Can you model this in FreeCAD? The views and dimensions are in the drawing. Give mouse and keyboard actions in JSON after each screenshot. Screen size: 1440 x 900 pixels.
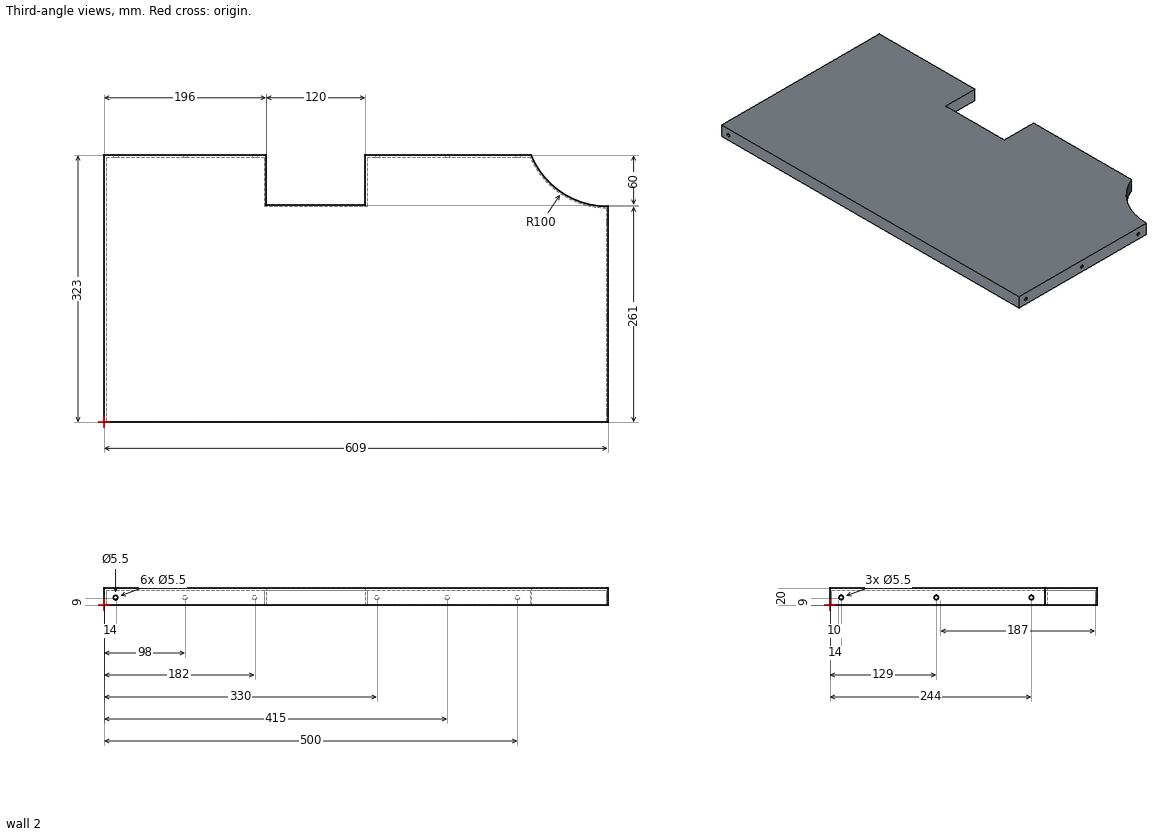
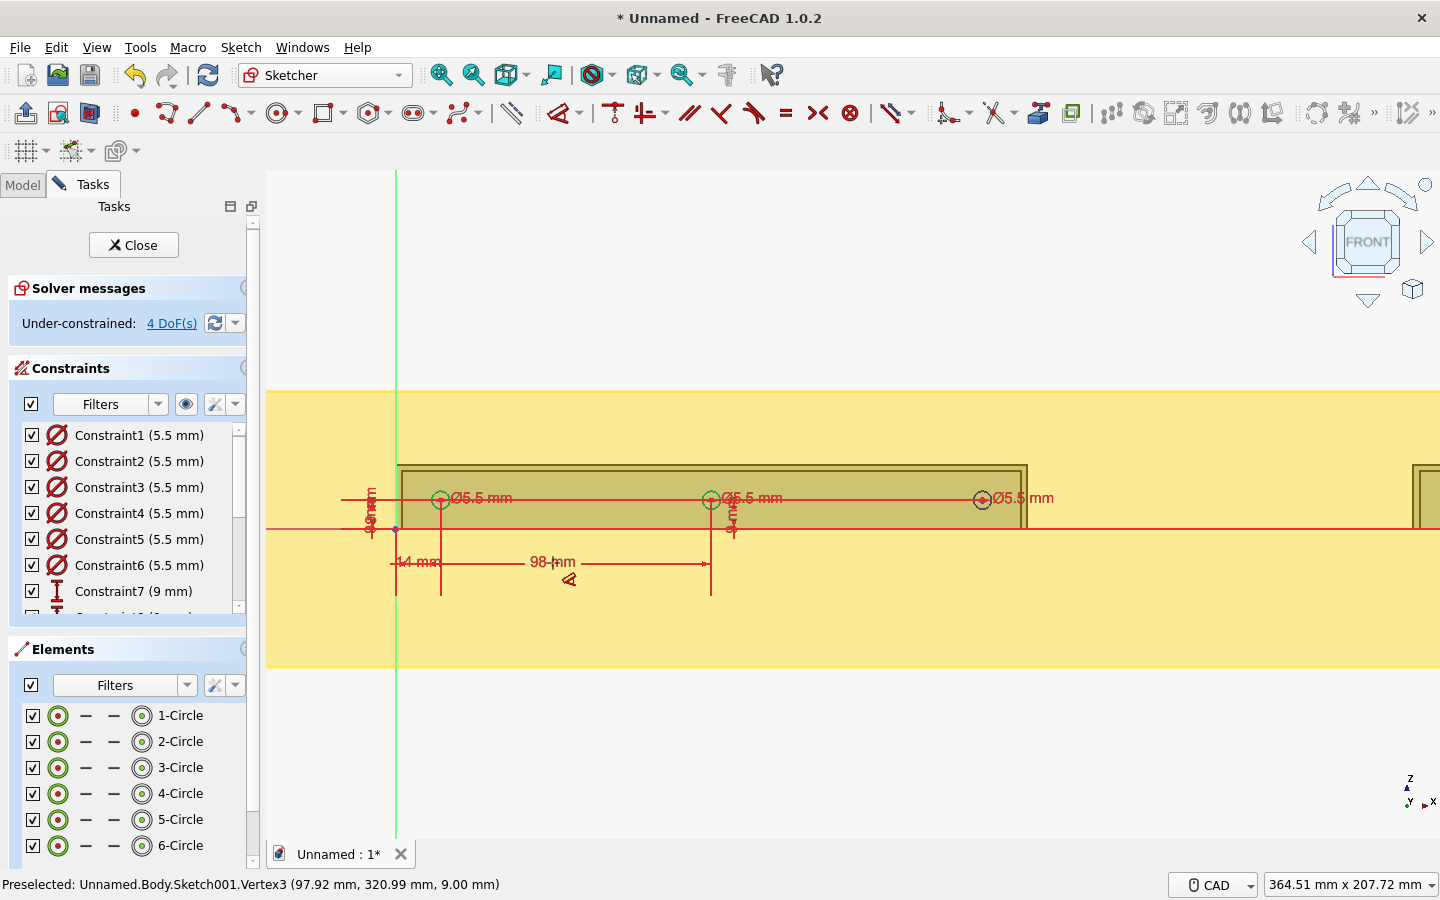
{"action": "left_click", "coordinate": [983, 500]}
{"action": "left_click", "coordinate": [689, 563]}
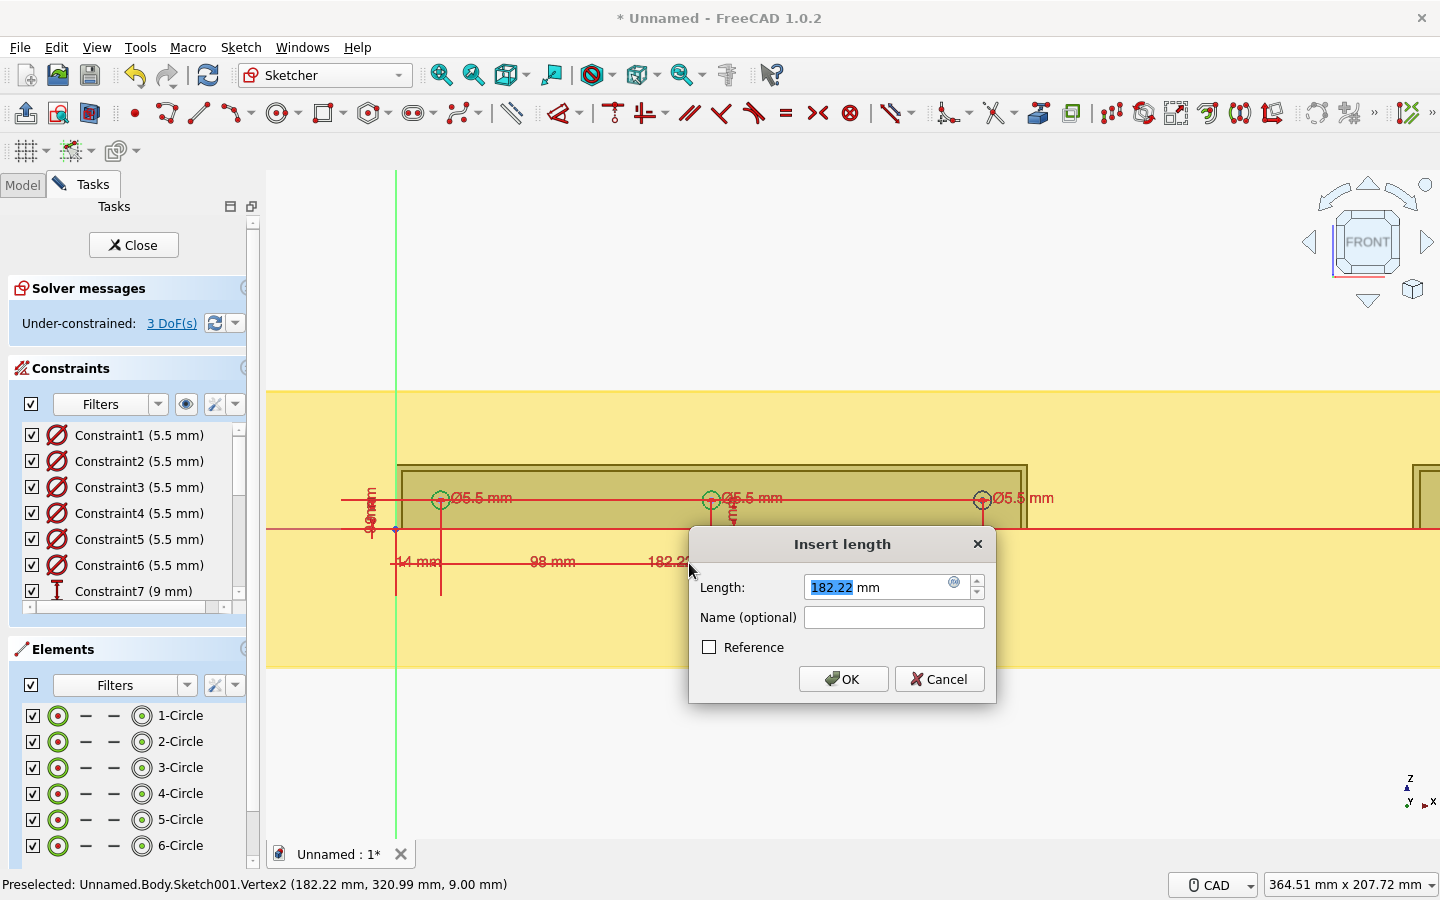
{"action": "type", "text": "182"}
{"action": "key", "text": "Return"}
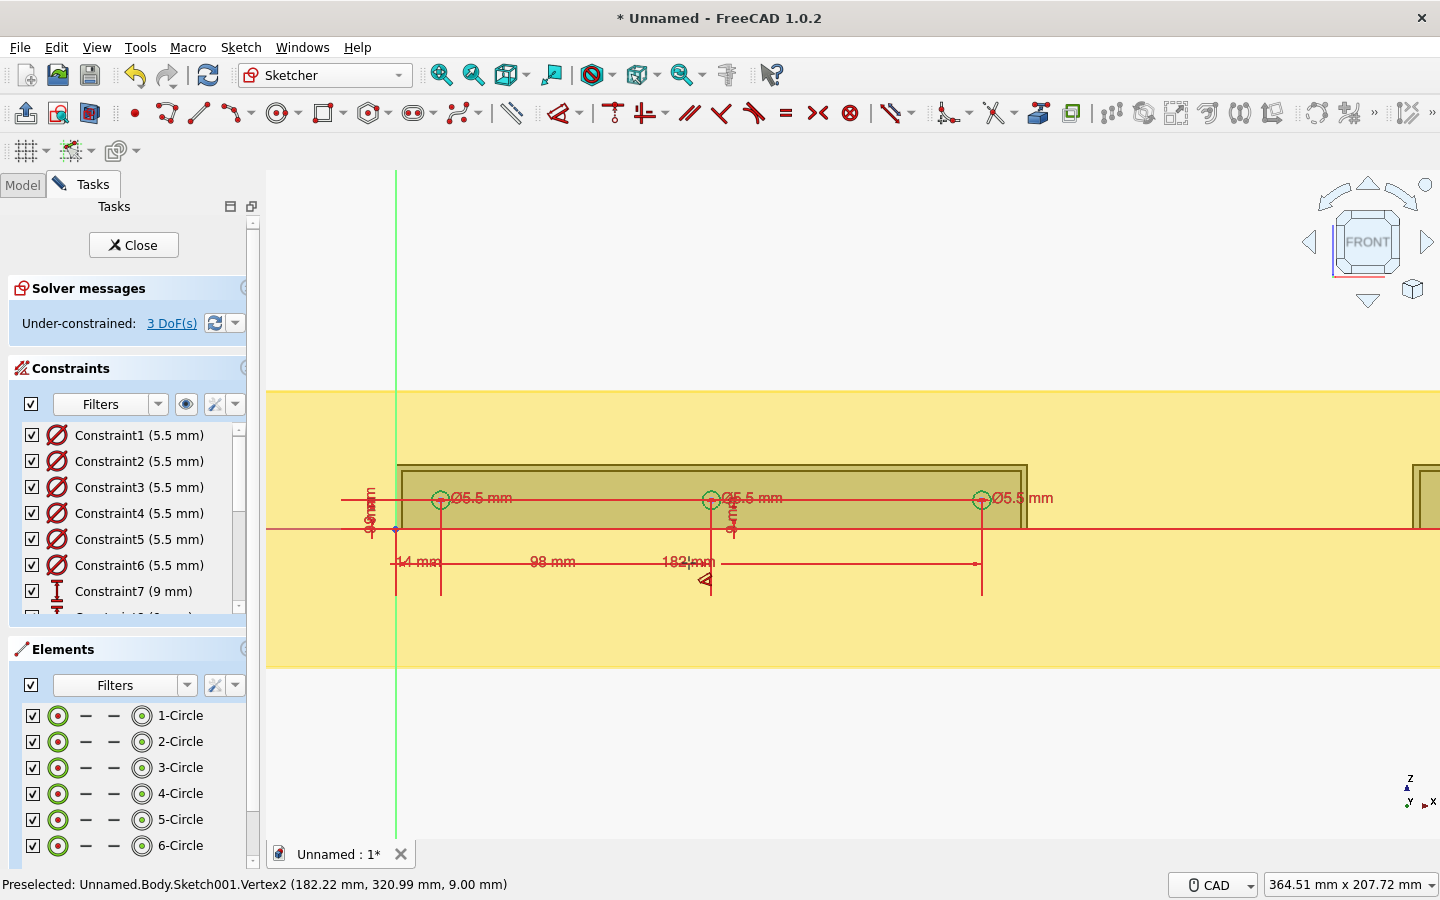
{"action": "scroll", "coordinate": [441, 500], "scroll_direction": "down", "scroll_amount": 4}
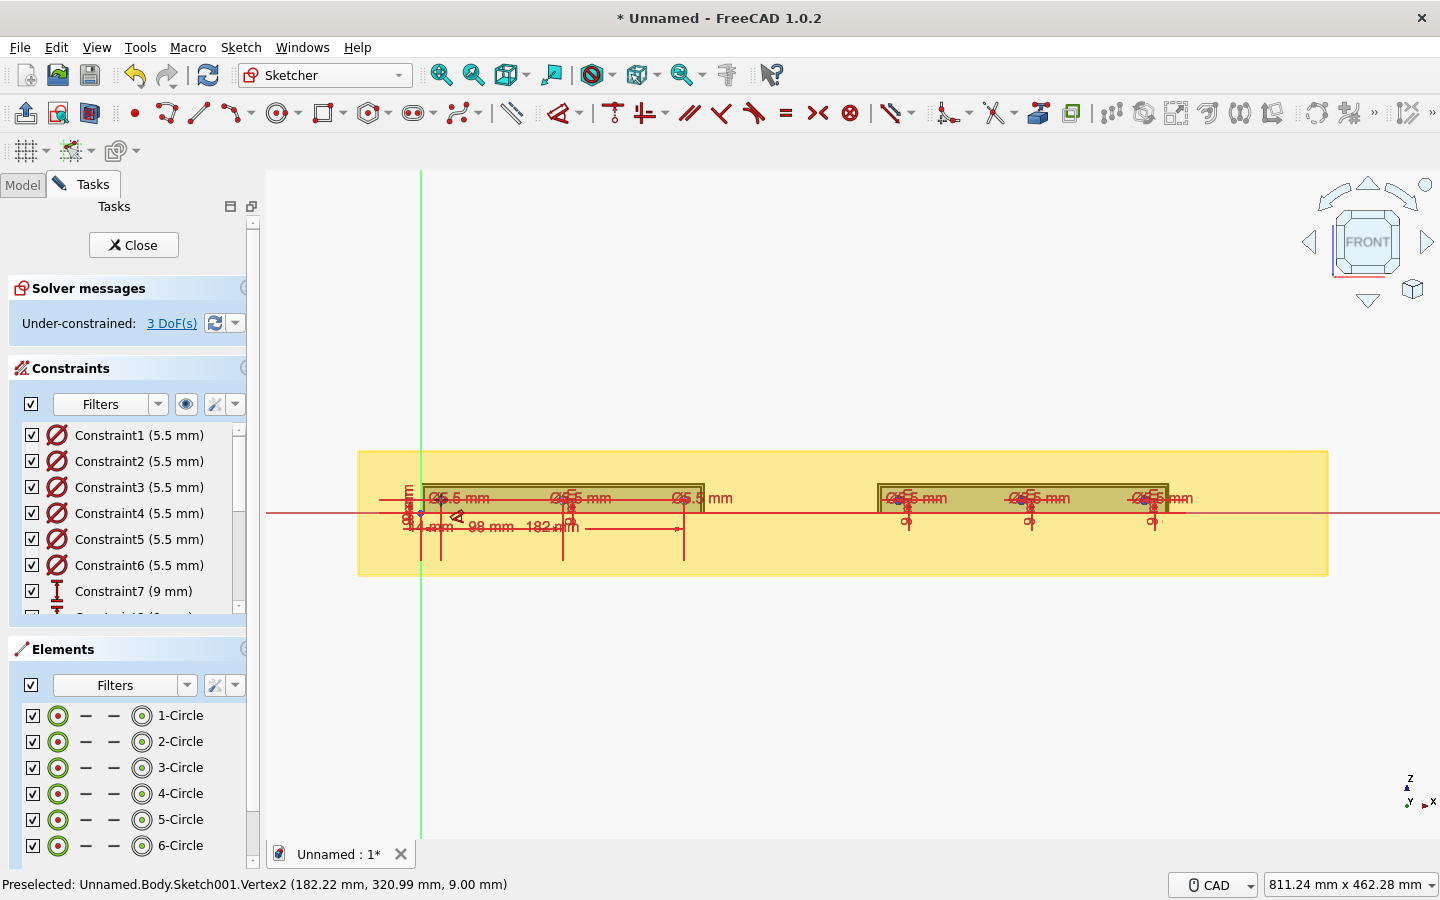
{"action": "left_click", "coordinate": [898, 500]}
{"action": "left_click", "coordinate": [660, 547]}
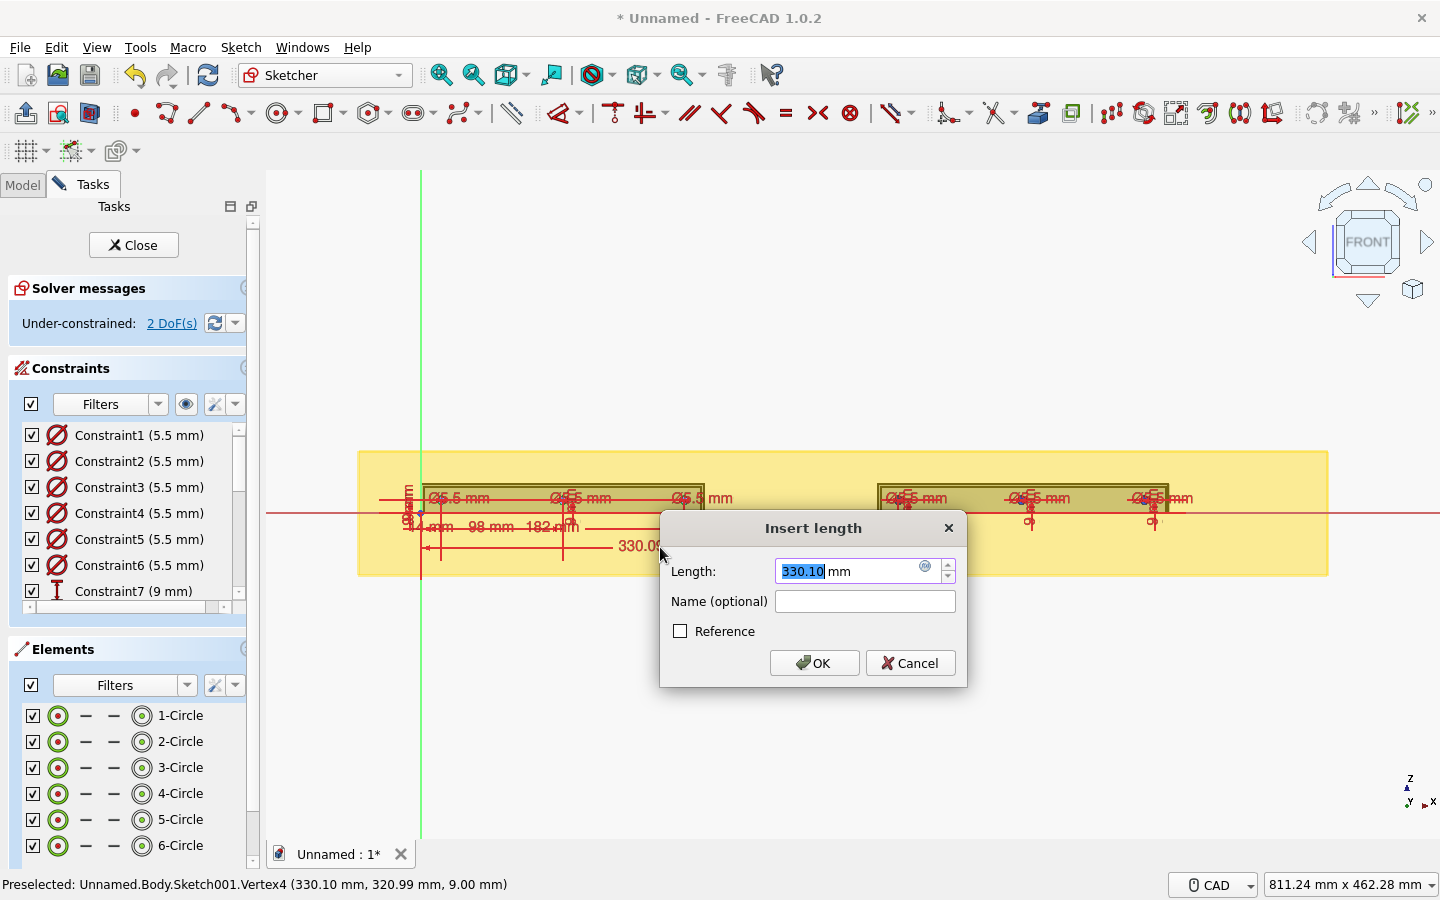
{"action": "type", "text": "330"}
{"action": "key", "text": "Return"}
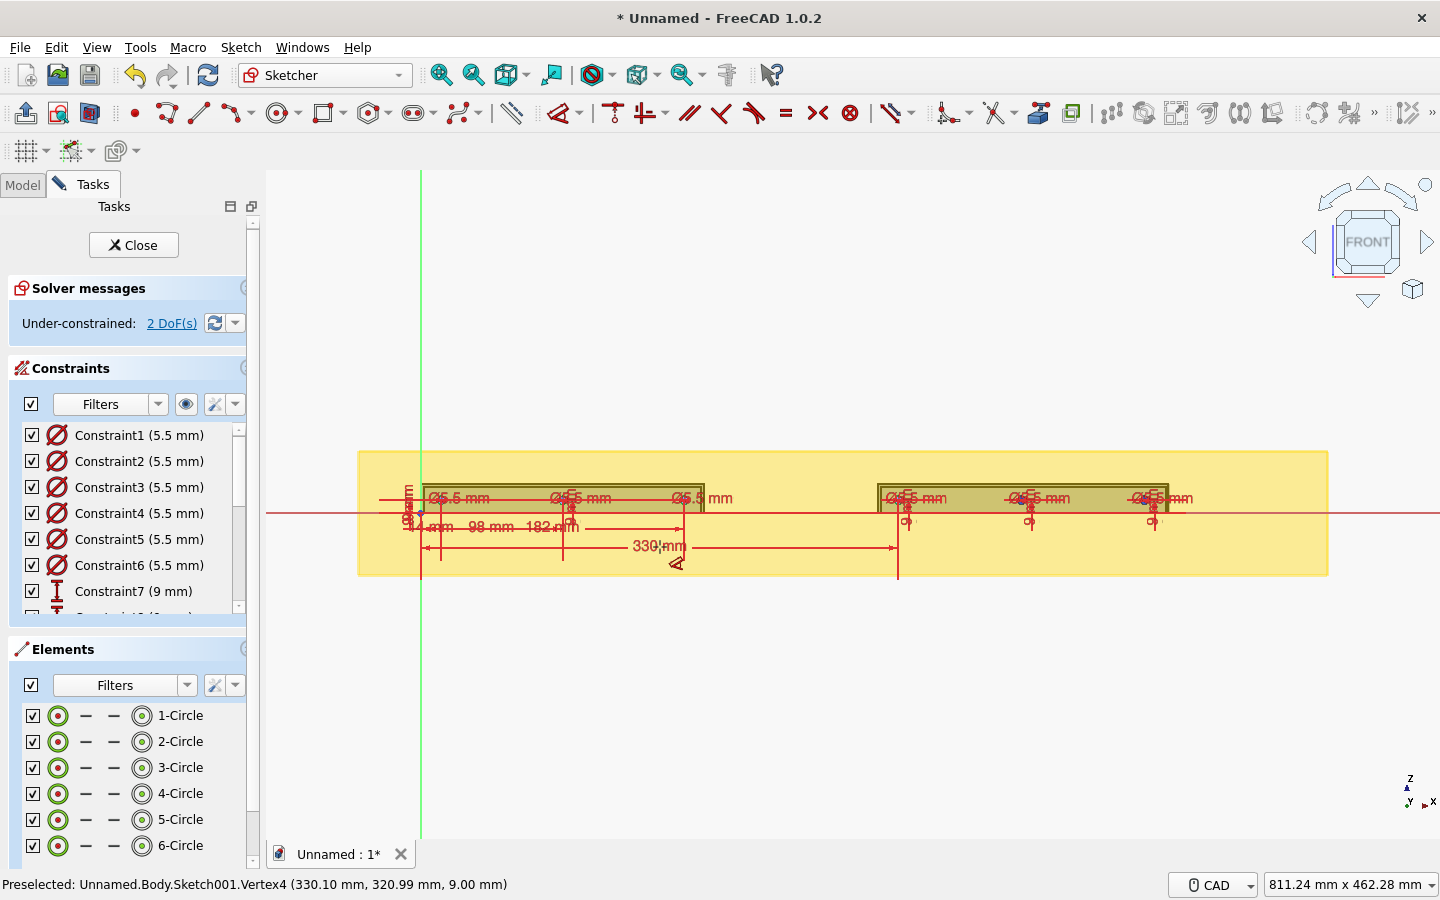
{"action": "left_click", "coordinate": [1144, 500]}
{"action": "left_click", "coordinate": [783, 547]}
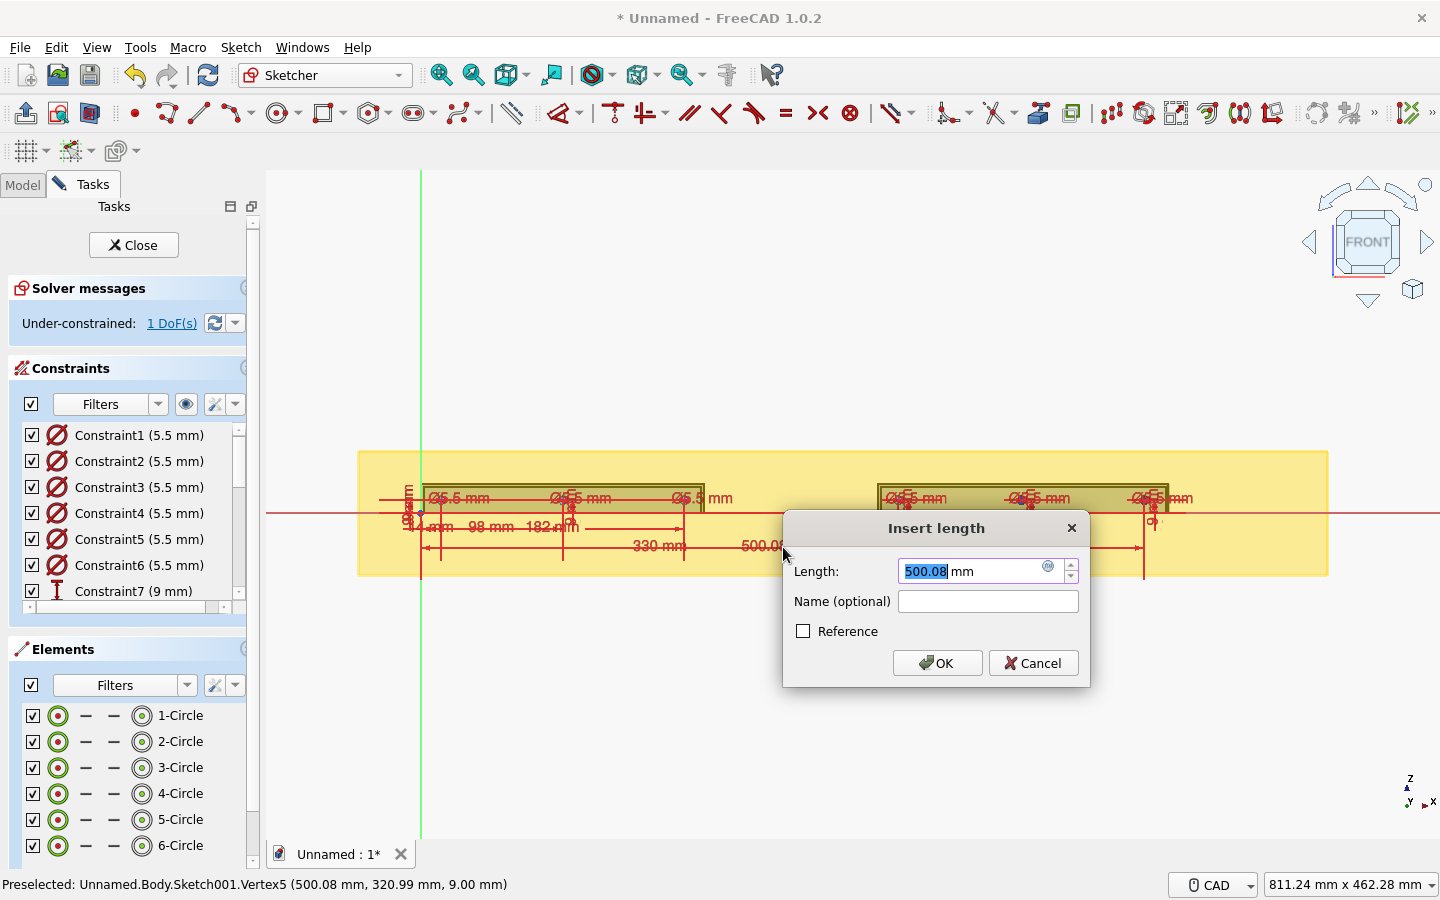
{"action": "type", "text": "500"}
{"action": "key", "text": "Return"}